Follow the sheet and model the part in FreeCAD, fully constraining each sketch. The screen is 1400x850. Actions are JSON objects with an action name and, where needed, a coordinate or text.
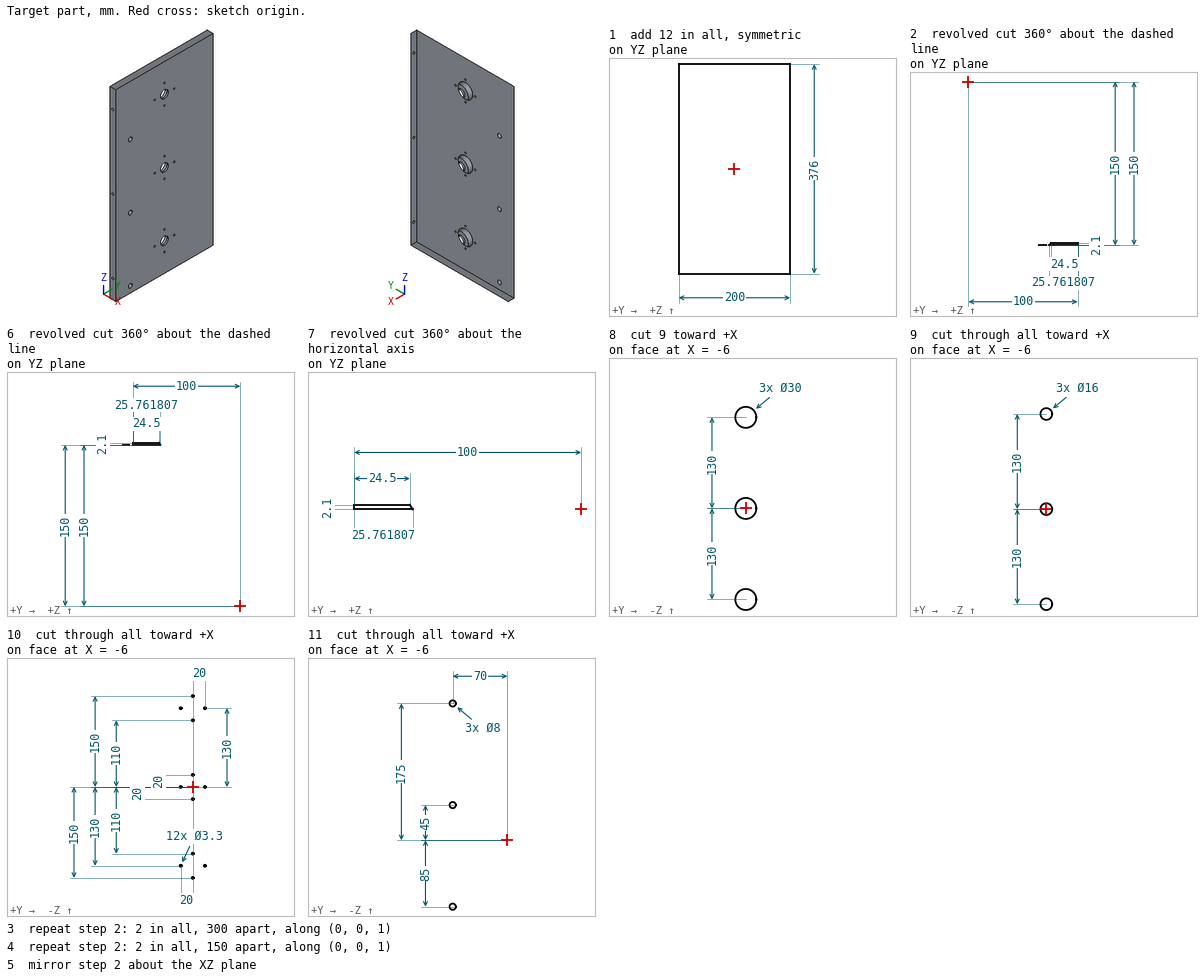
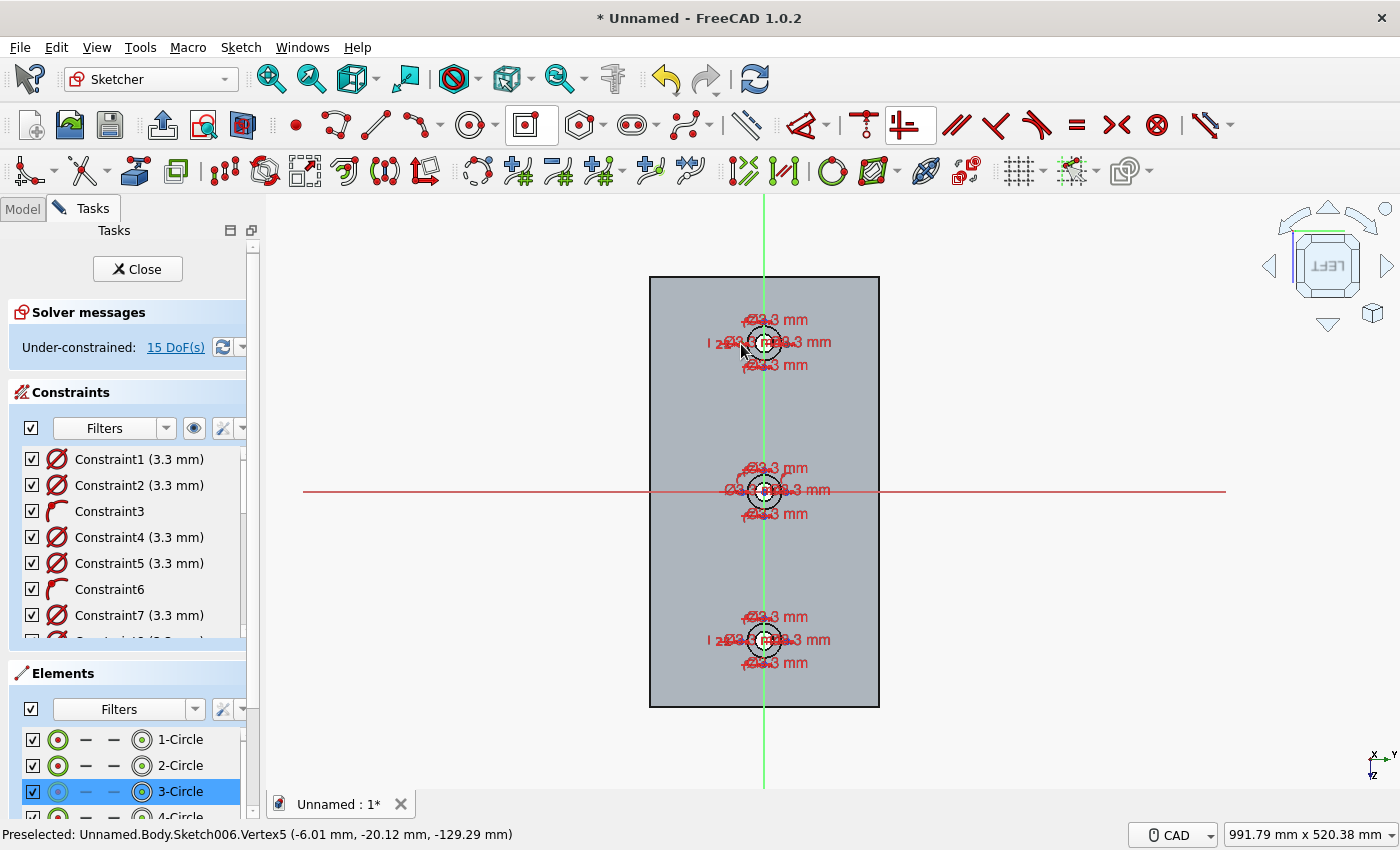
{"action": "left_click", "coordinate": [930, 126]}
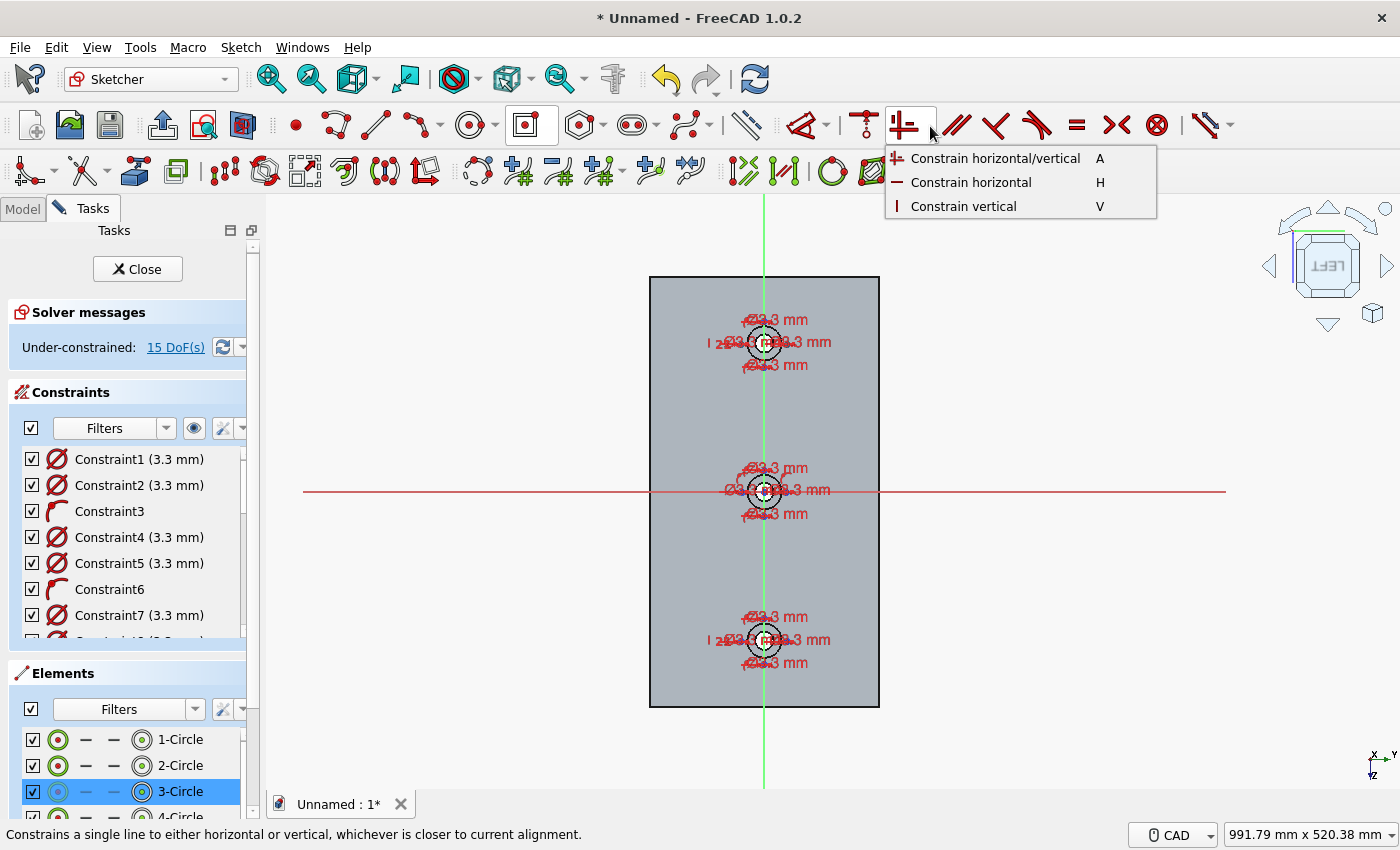
{"action": "left_click", "coordinate": [1021, 182]}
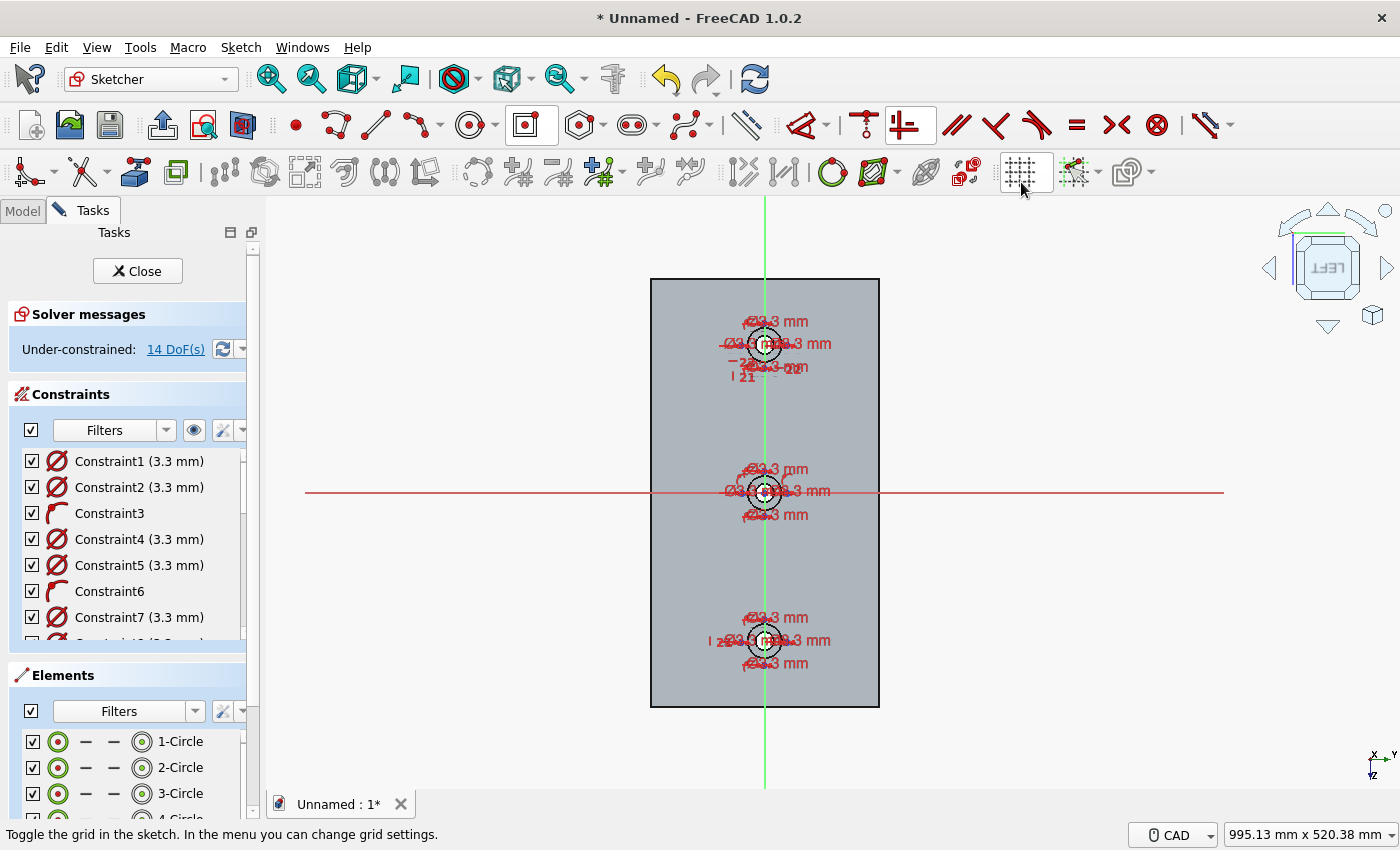
{"action": "left_click", "coordinate": [788, 346]}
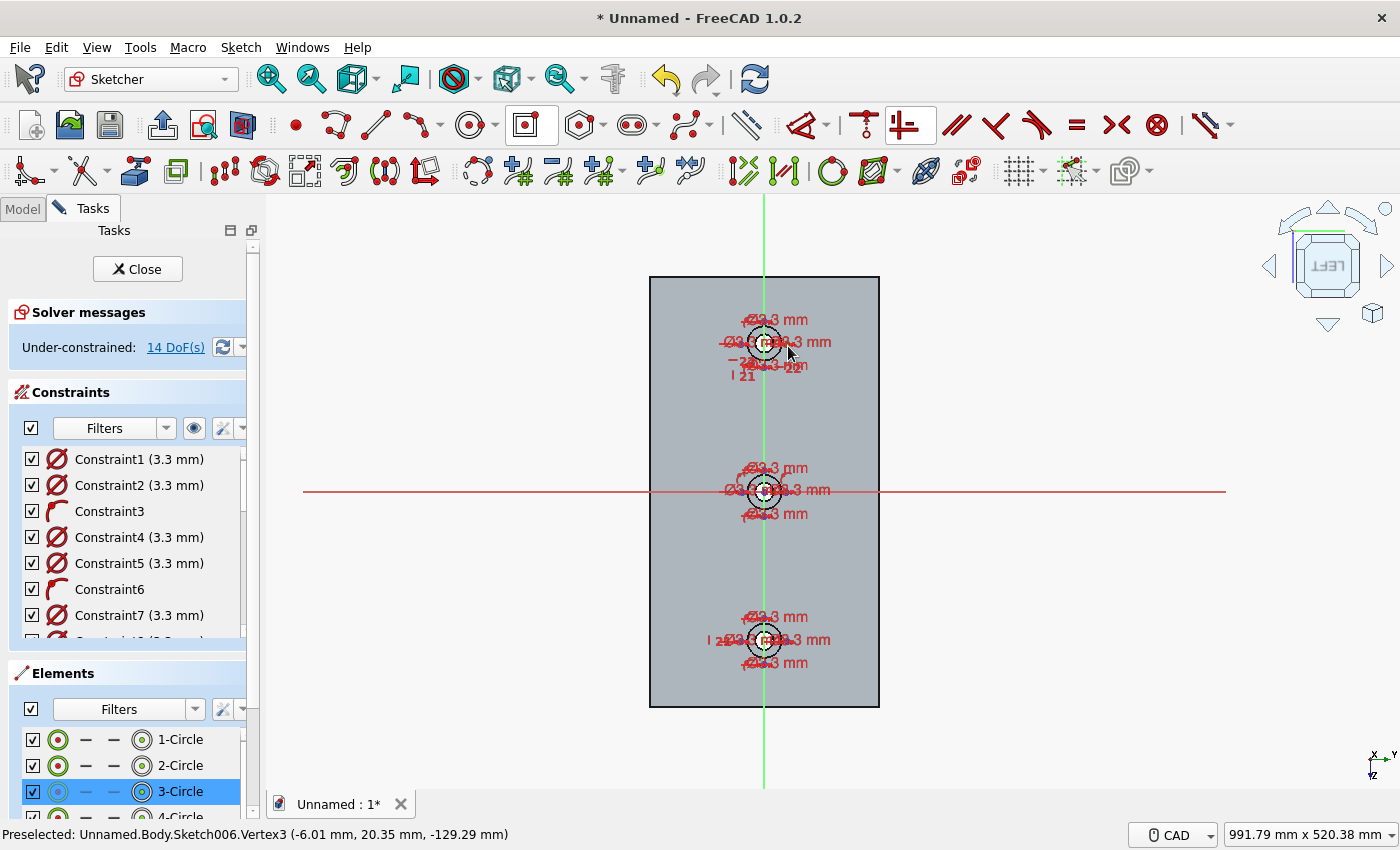
{"action": "left_click", "coordinate": [787, 492]}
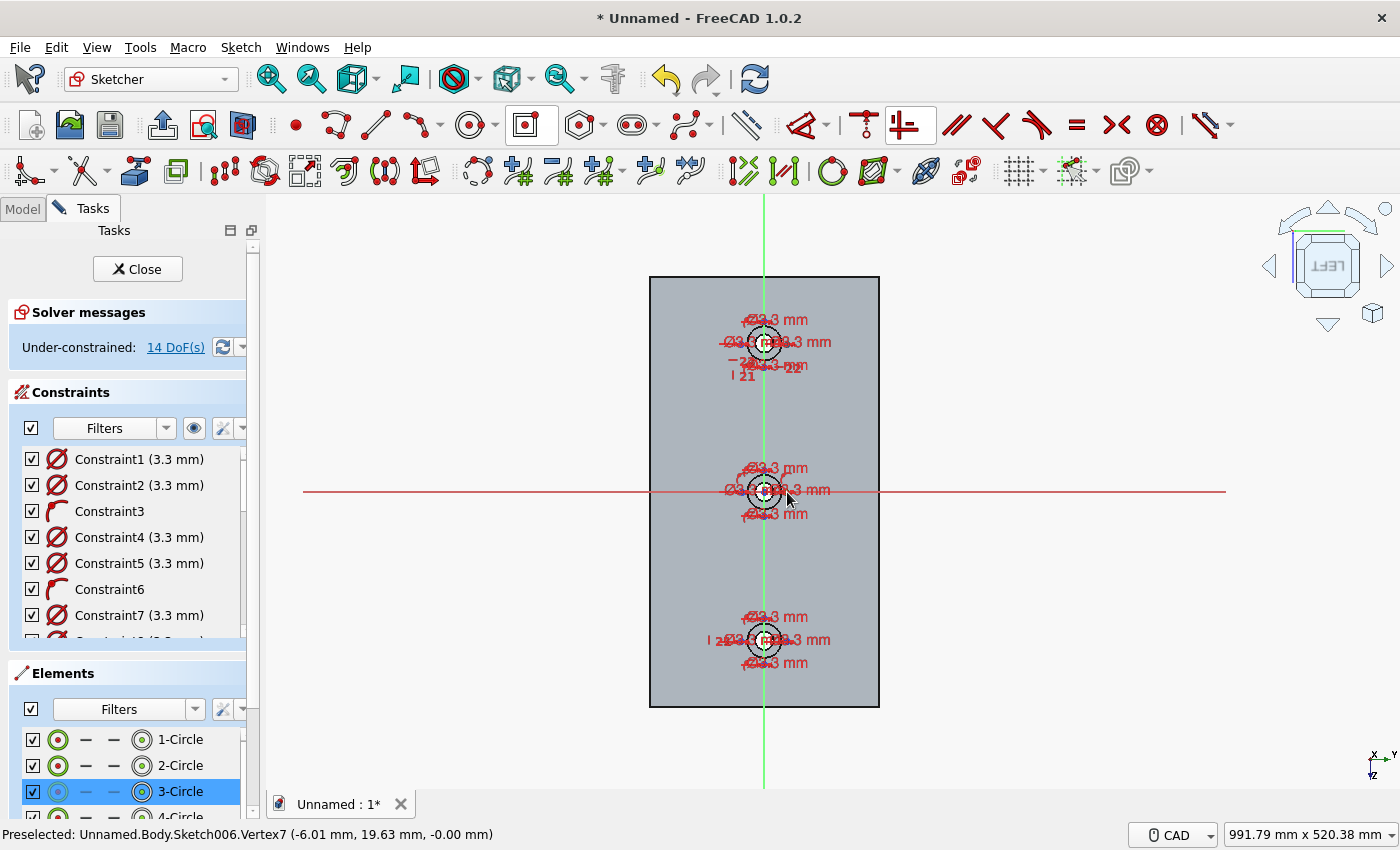
{"action": "left_click", "coordinate": [930, 126]}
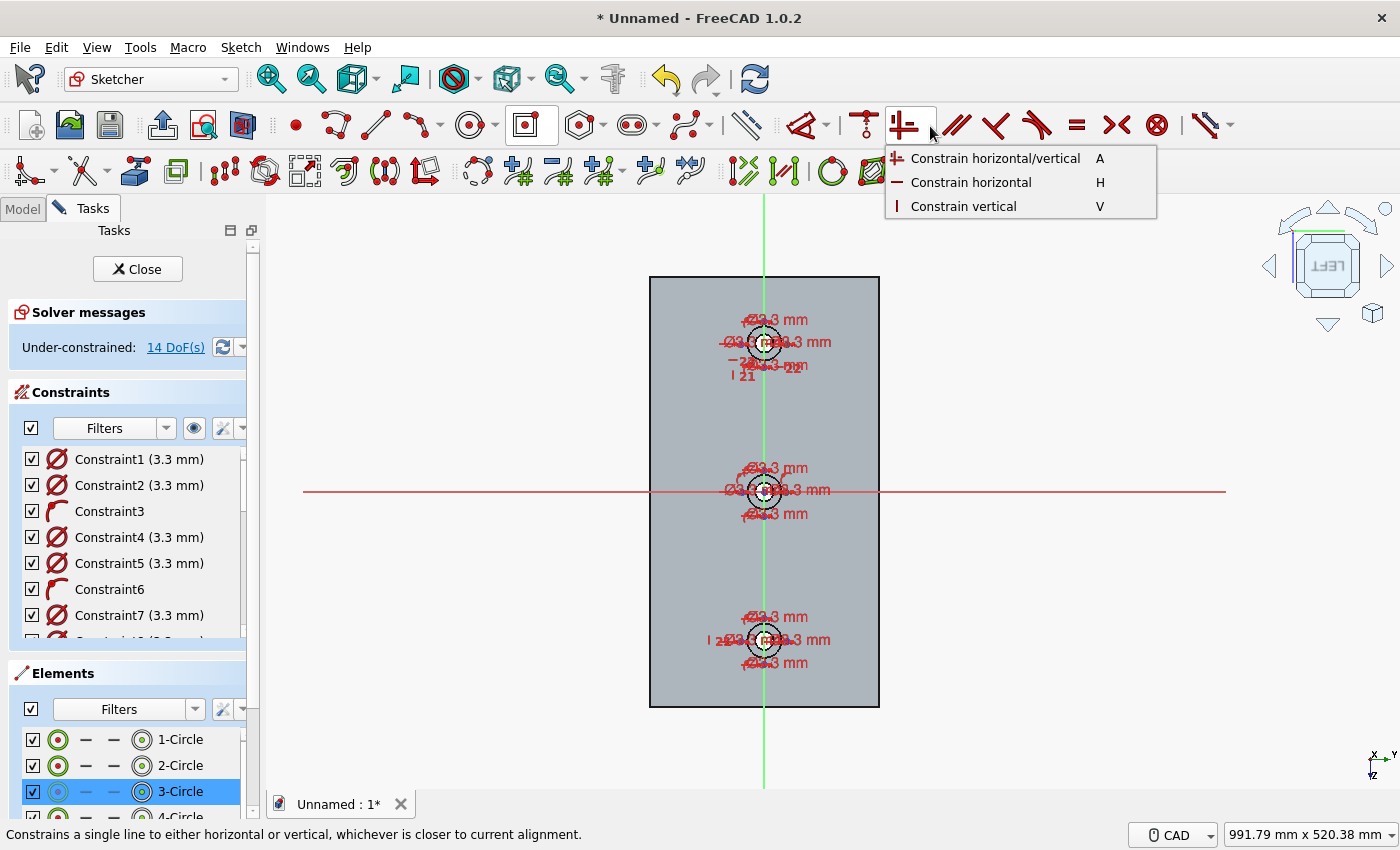
{"action": "left_click", "coordinate": [1021, 206]}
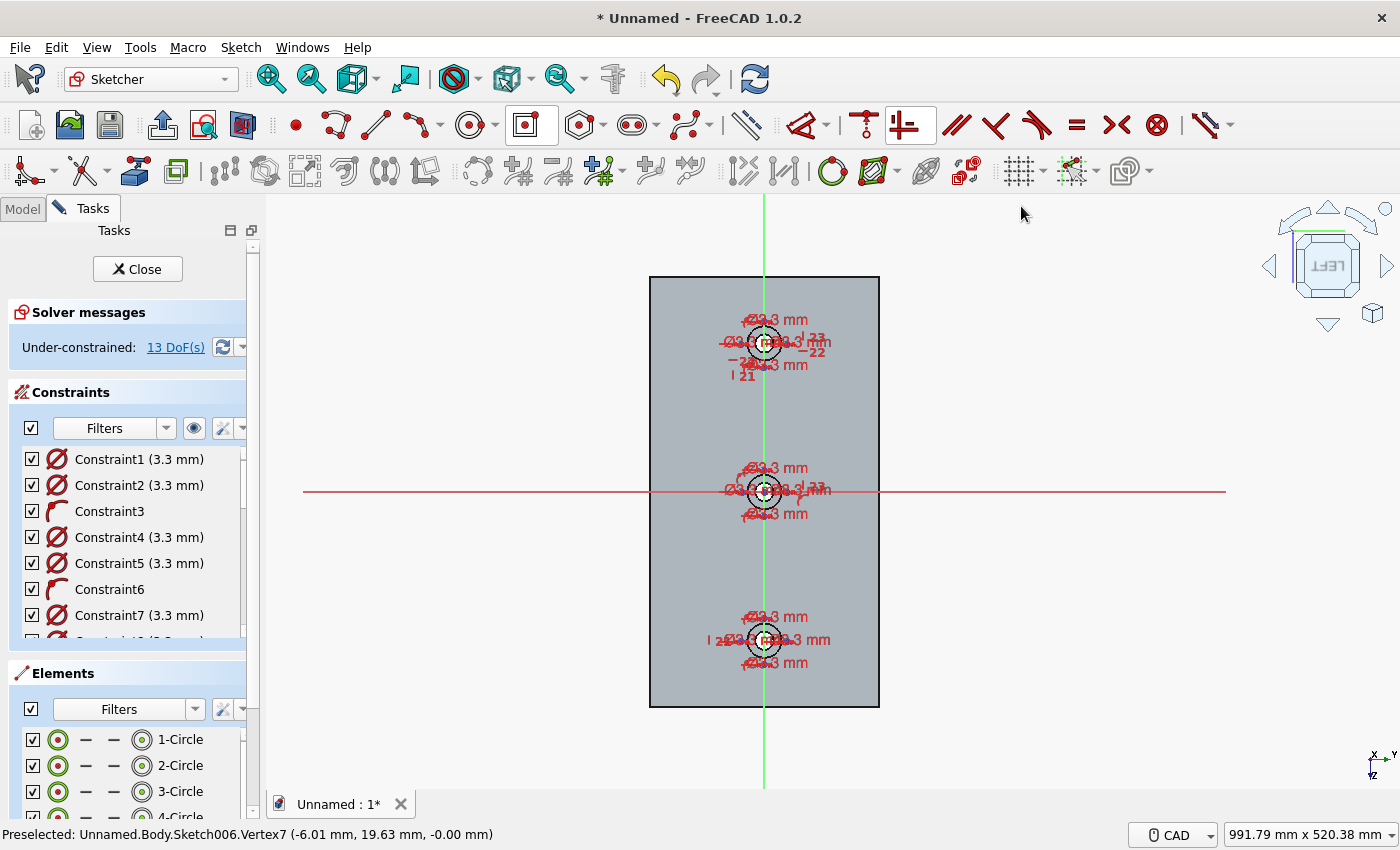
{"action": "left_click", "coordinate": [741, 642]}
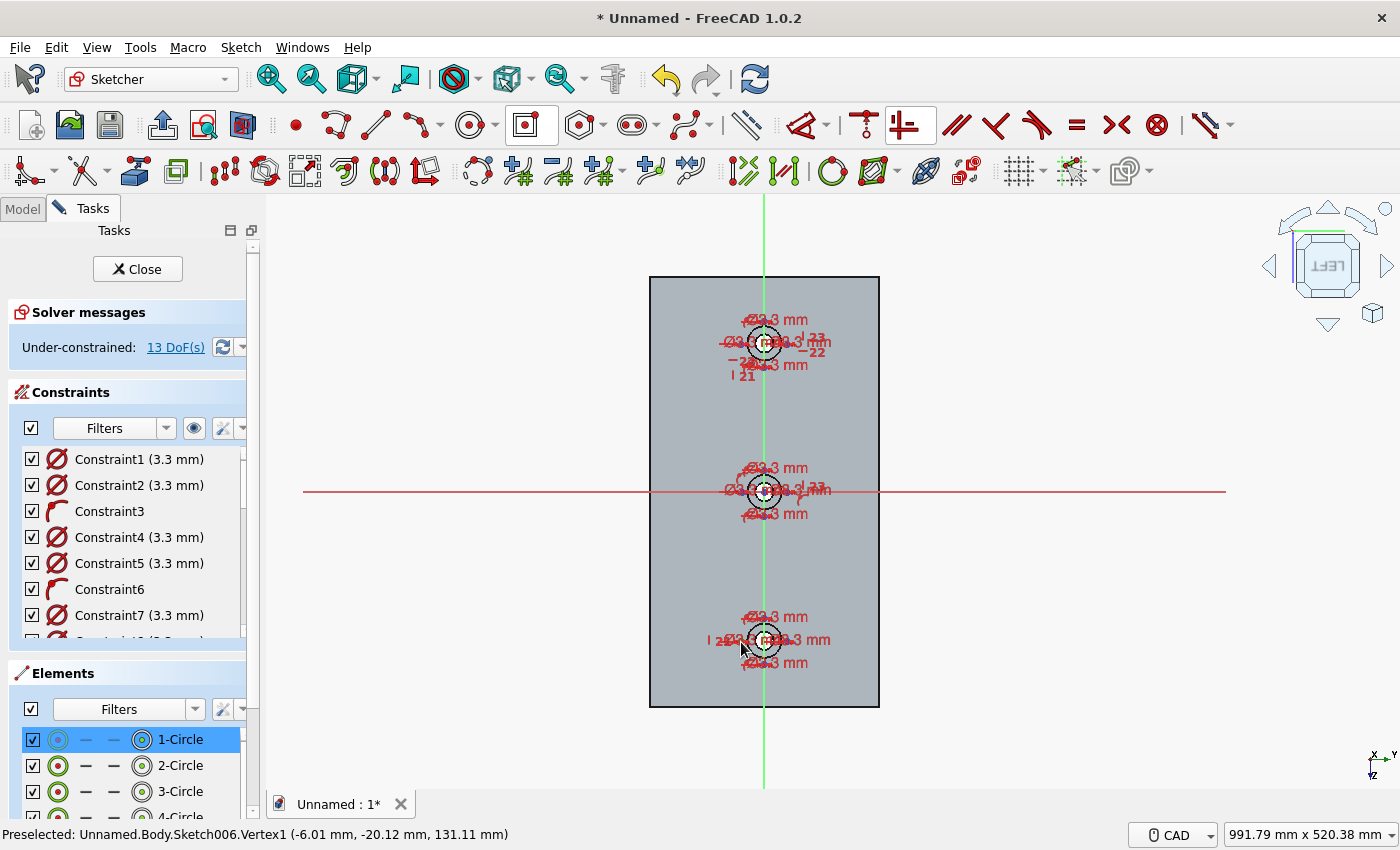
{"action": "left_click", "coordinate": [742, 492]}